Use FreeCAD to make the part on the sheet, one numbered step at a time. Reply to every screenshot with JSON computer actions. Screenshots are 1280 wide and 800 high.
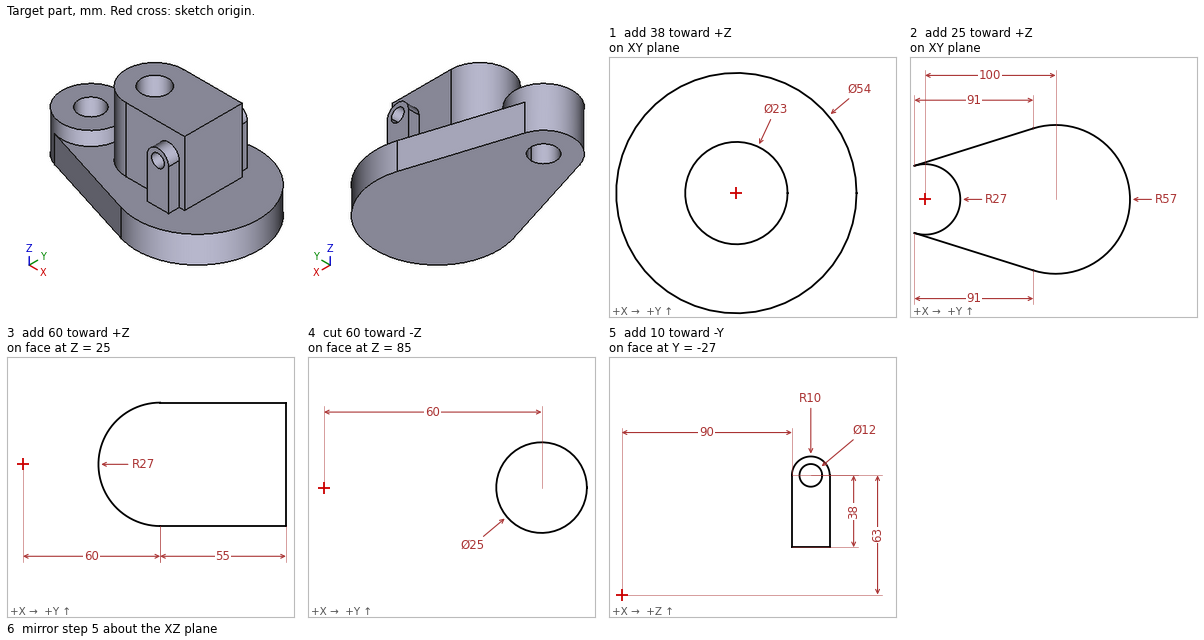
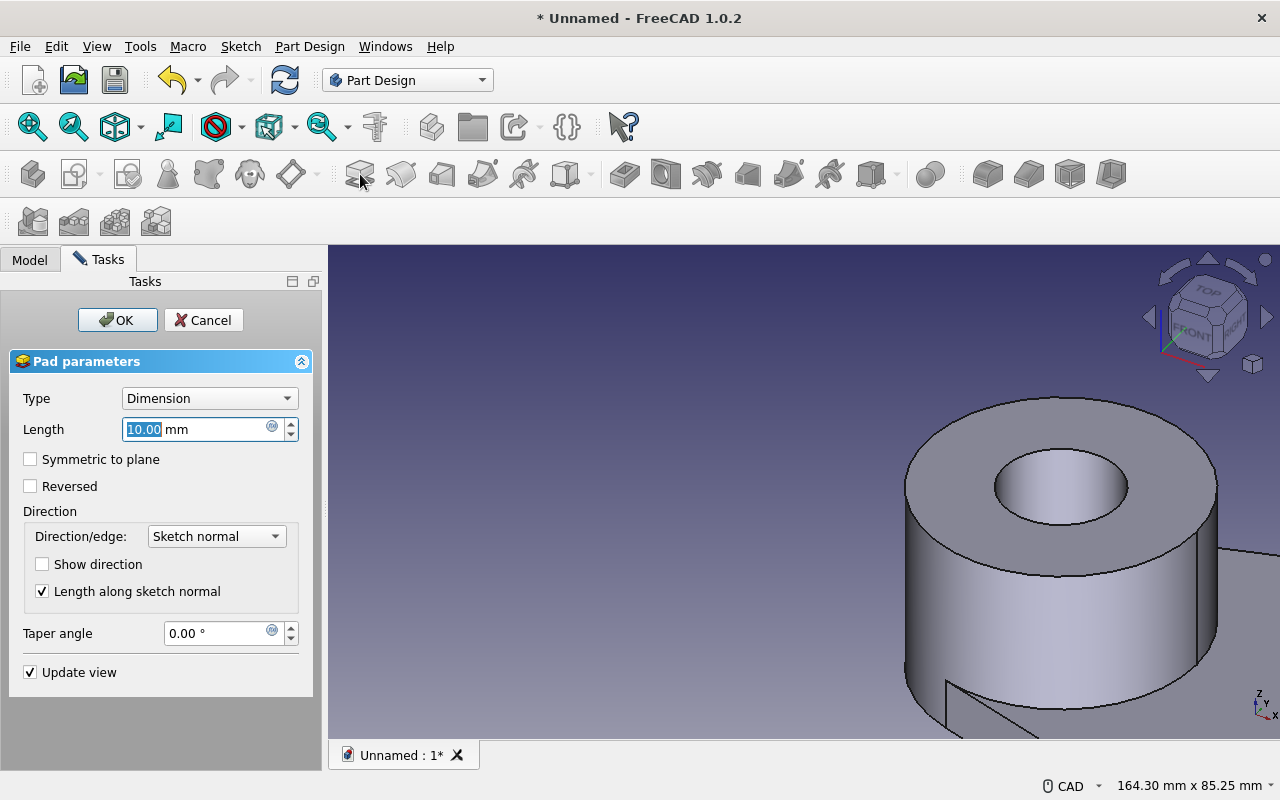
{"action": "type", "text": "25"}
{"action": "key", "text": "Tab"}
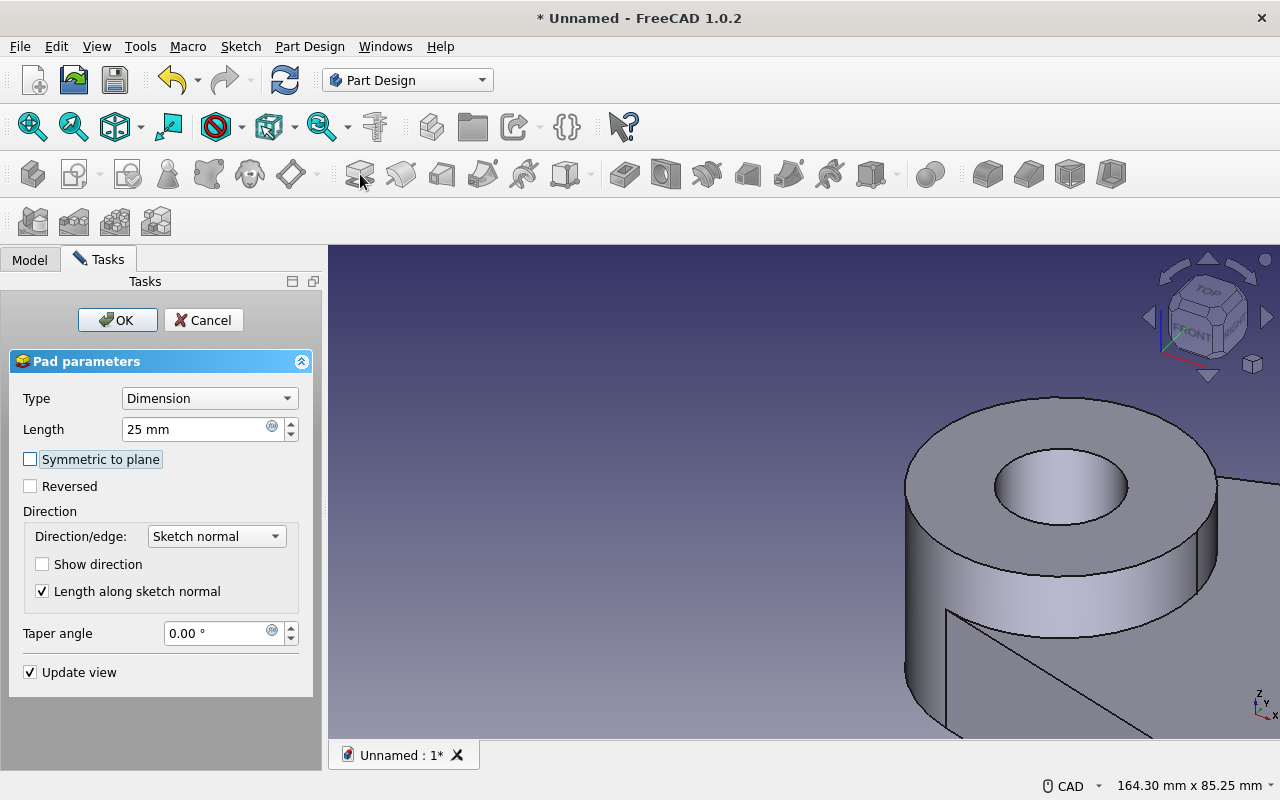
{"action": "left_click", "coordinate": [118, 320]}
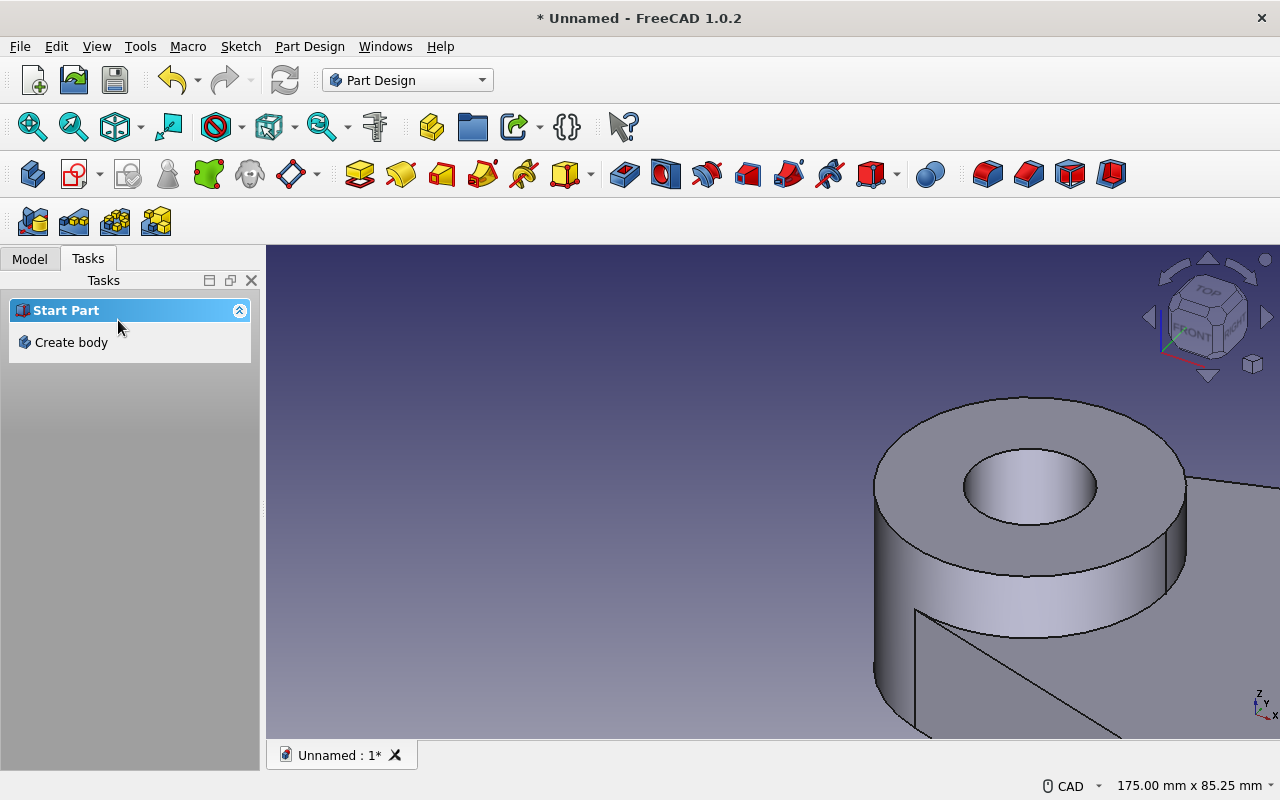
{"action": "left_click", "coordinate": [33, 128]}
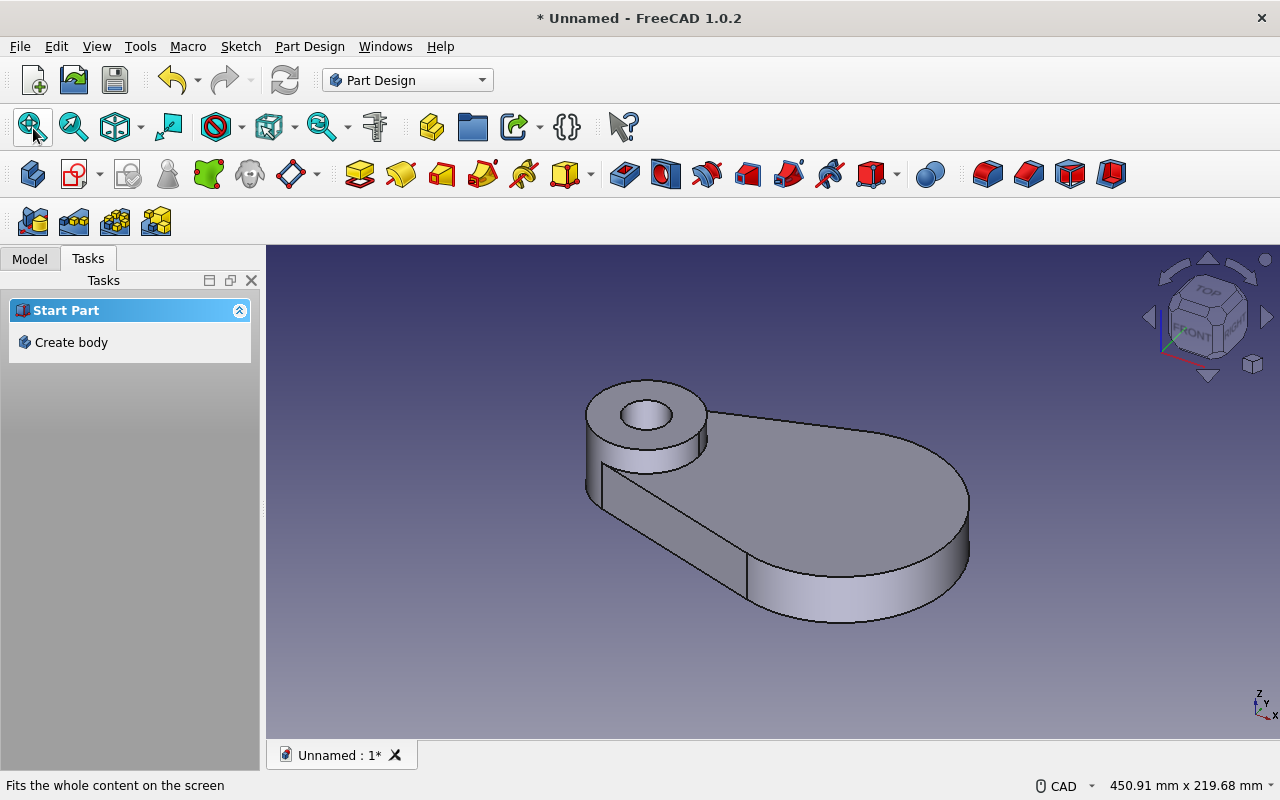
{"action": "left_click", "coordinate": [837, 501]}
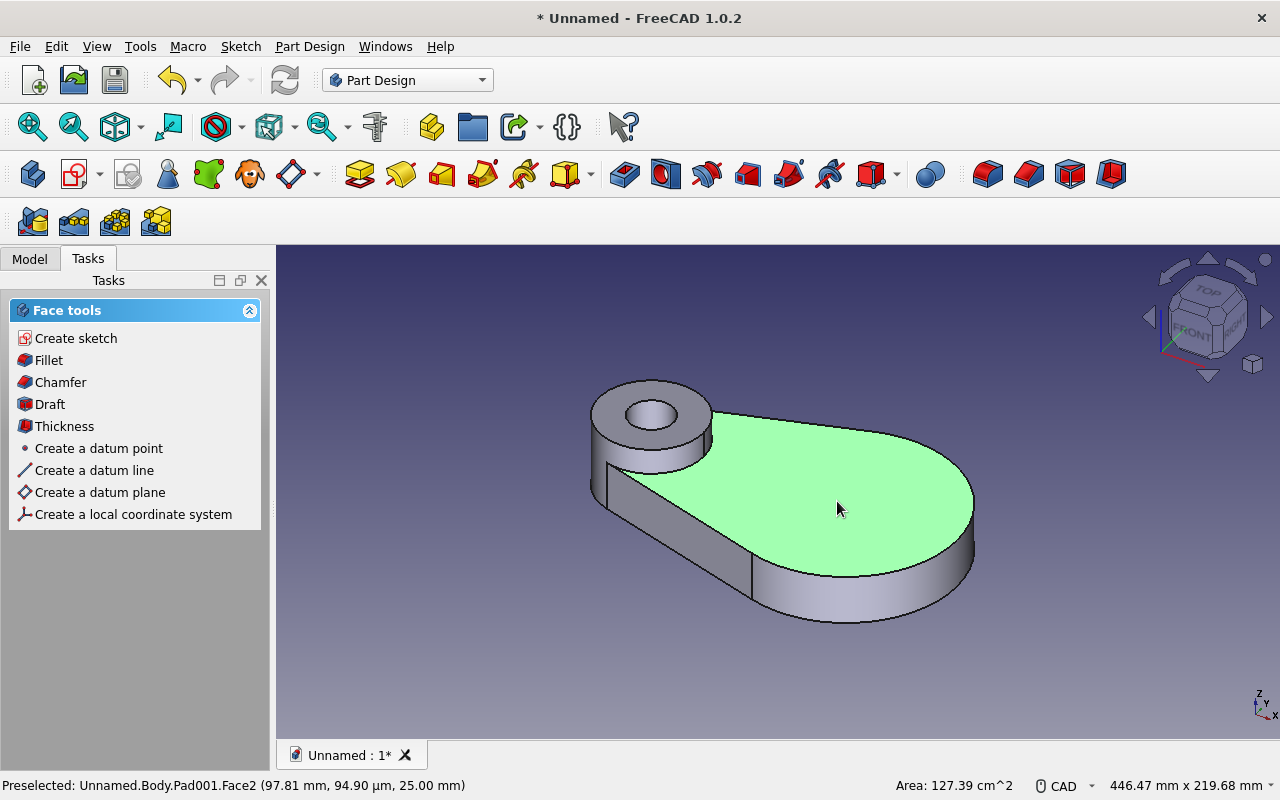
{"action": "left_click", "coordinate": [74, 174]}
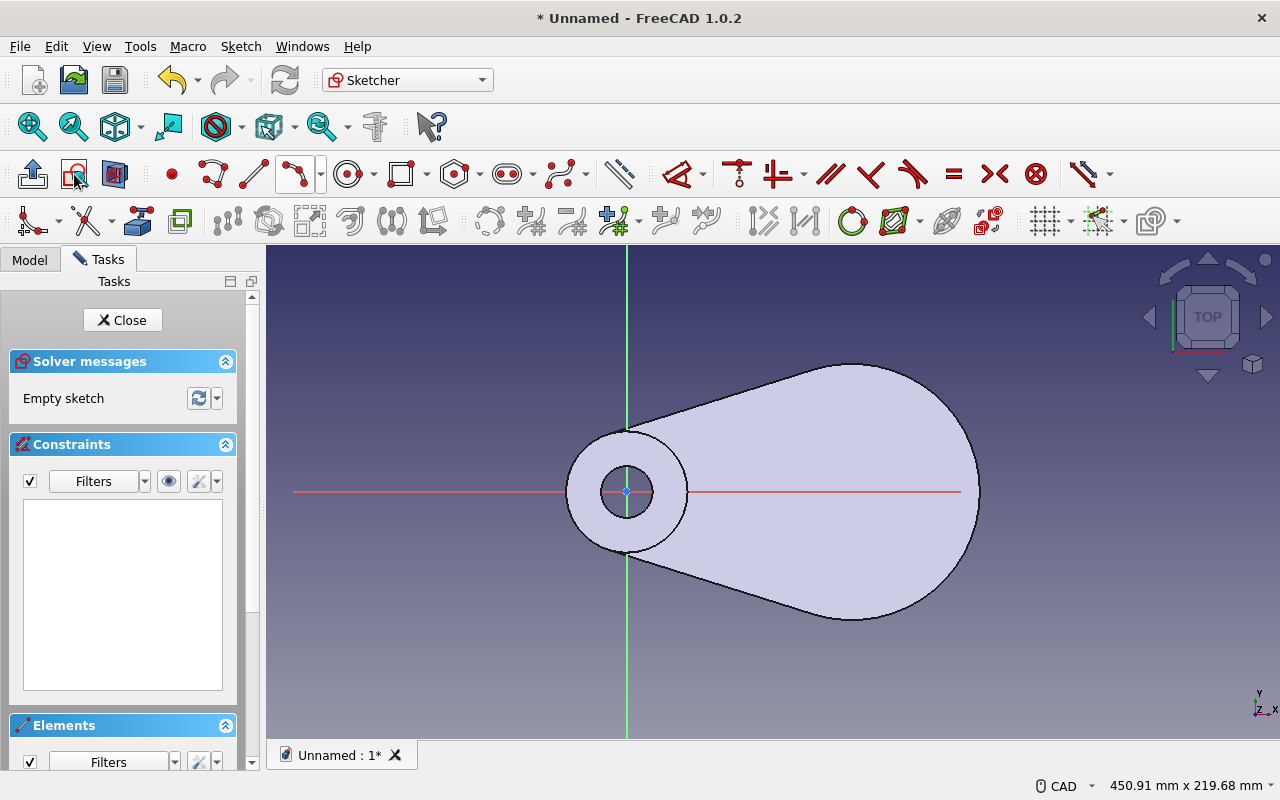
{"action": "scroll", "coordinate": [798, 492], "scroll_direction": "up", "scroll_amount": 4}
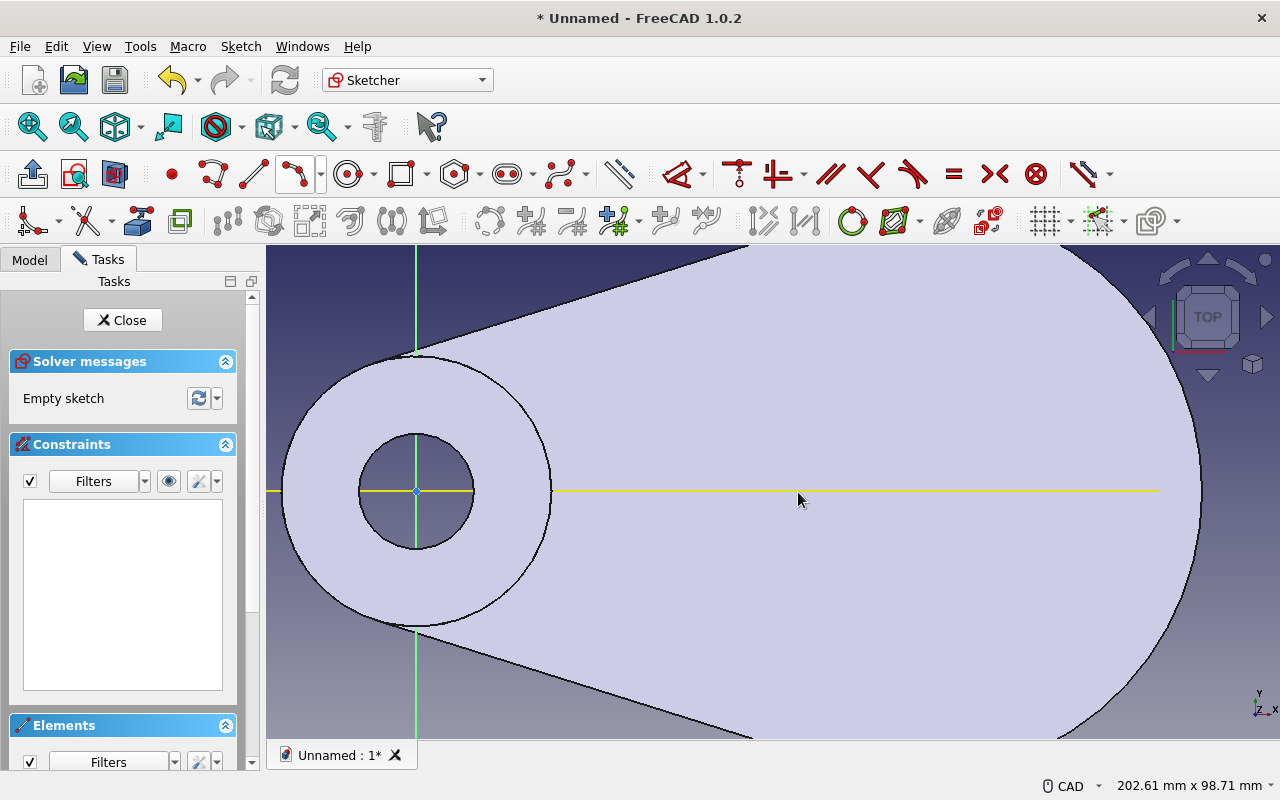
{"action": "key", "text": "g m"}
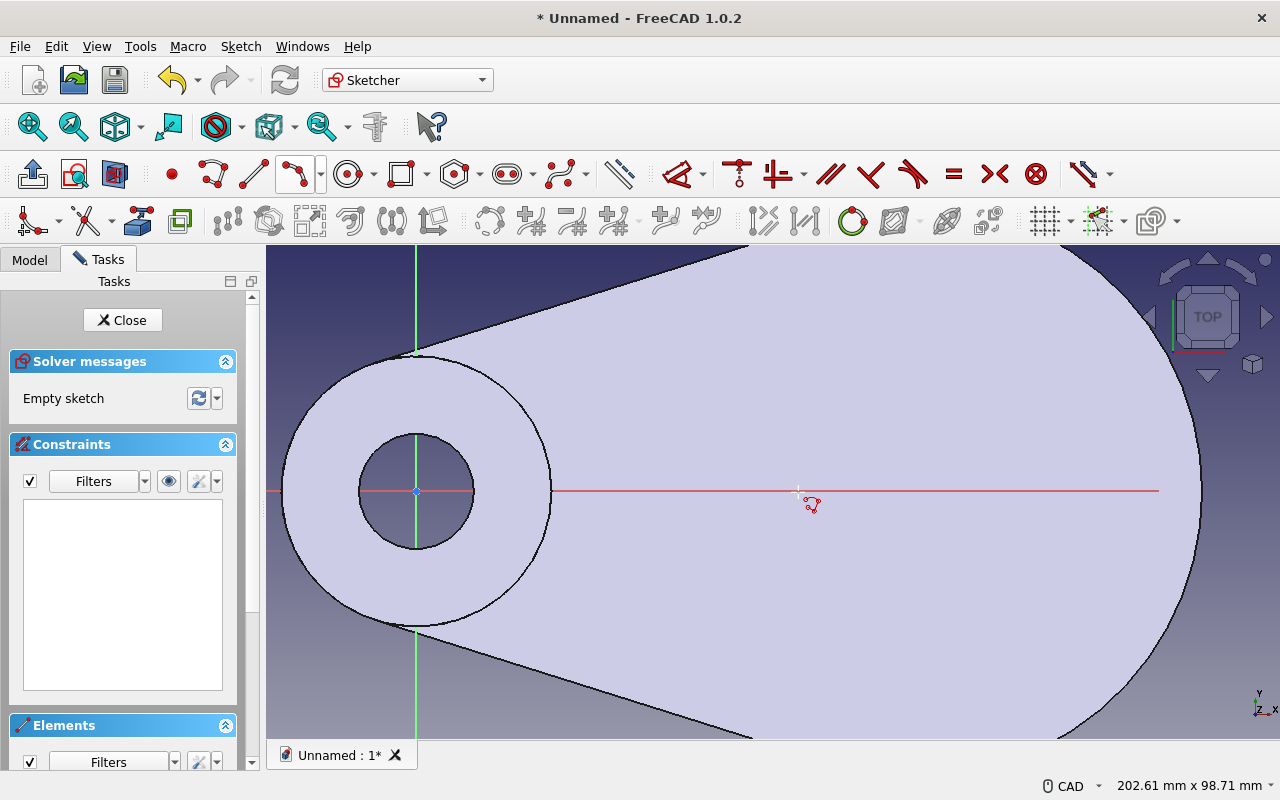
{"action": "left_click", "coordinate": [717, 627]}
{"action": "left_click", "coordinate": [992, 627]}
{"action": "left_click", "coordinate": [992, 356]}
{"action": "left_click", "coordinate": [717, 356]}
{"action": "right_click", "coordinate": [717, 356]}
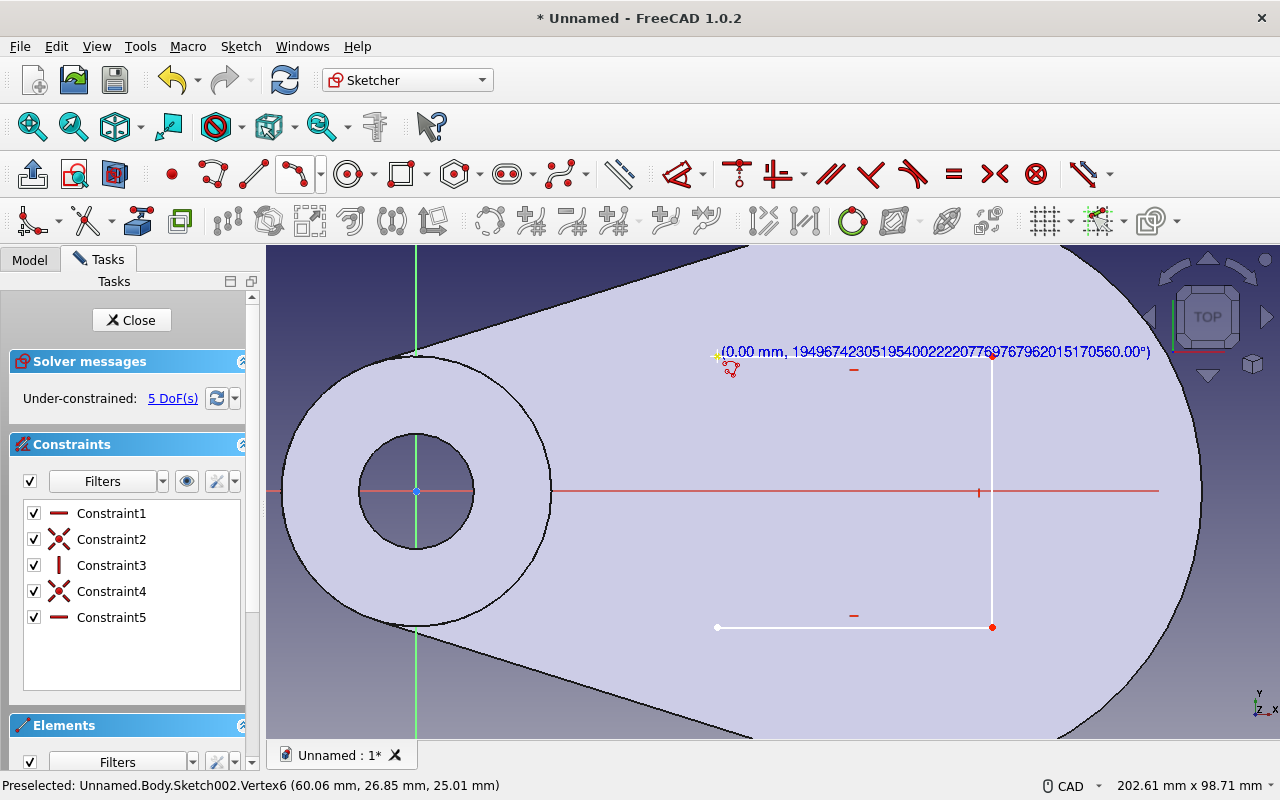
{"action": "key", "text": "g 3 a"}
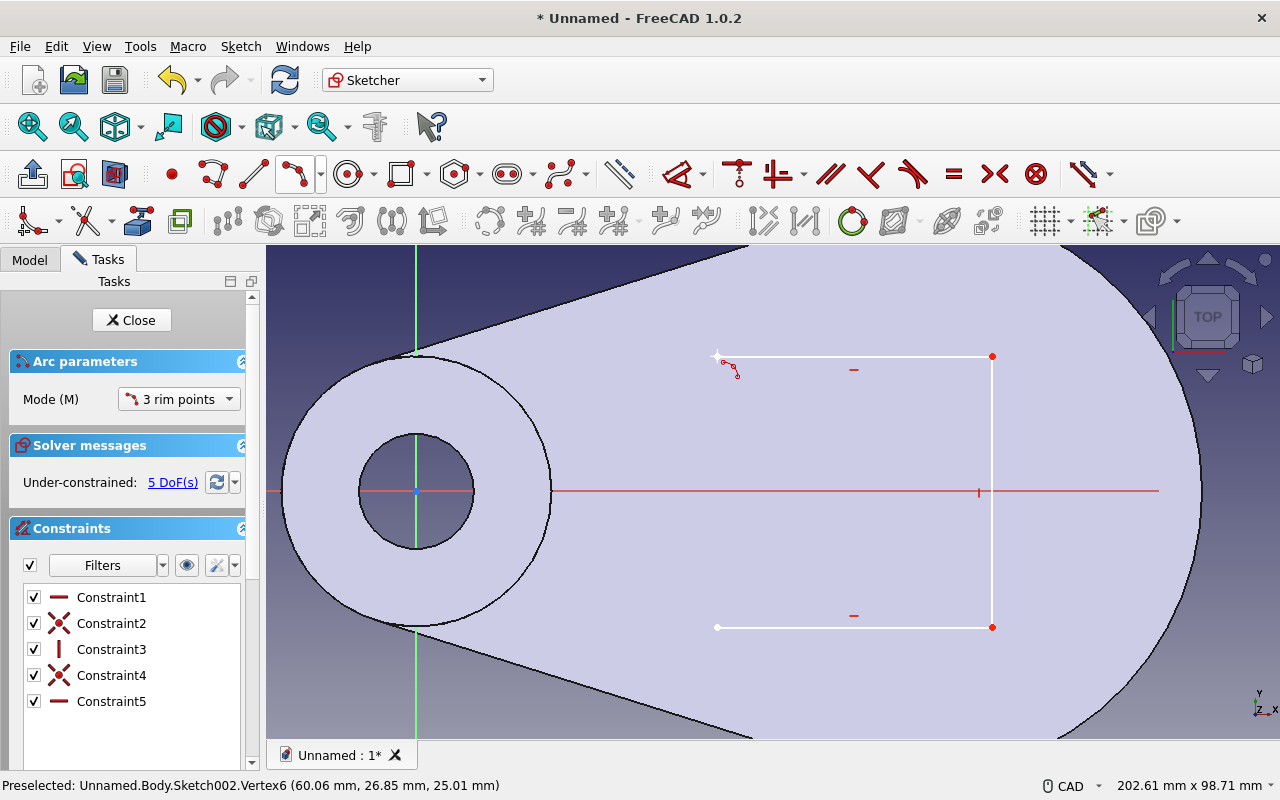
{"action": "left_click", "coordinate": [717, 357]}
{"action": "left_click", "coordinate": [717, 628]}
{"action": "left_click", "coordinate": [588, 450]}
{"action": "key", "text": "Escape"}